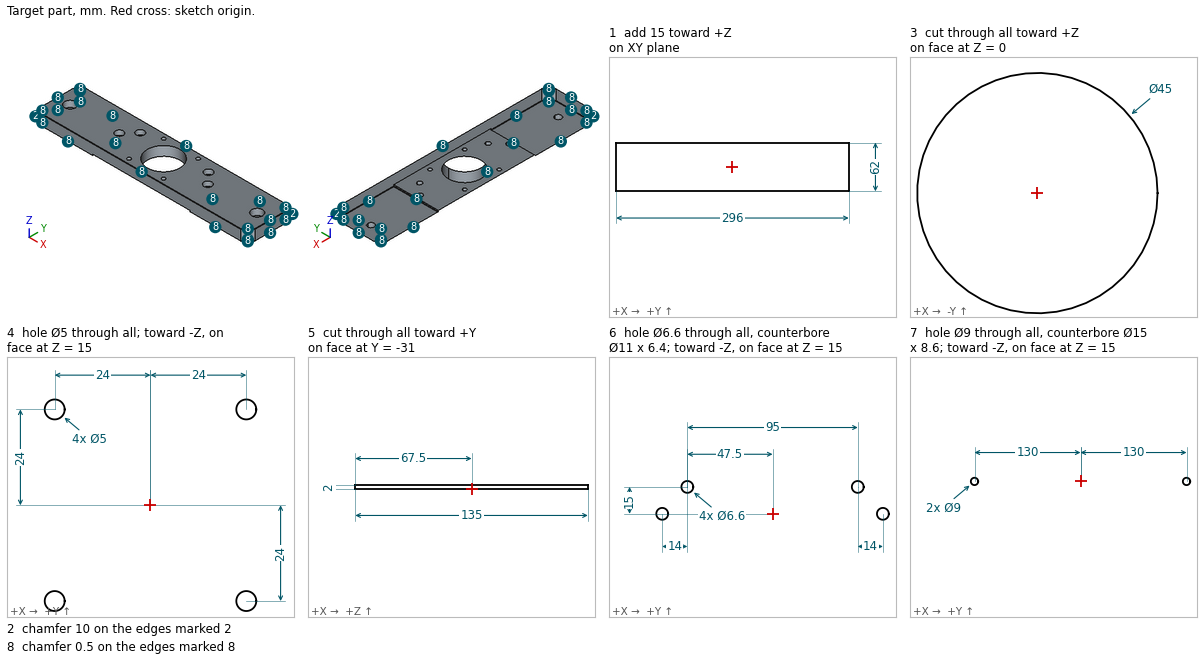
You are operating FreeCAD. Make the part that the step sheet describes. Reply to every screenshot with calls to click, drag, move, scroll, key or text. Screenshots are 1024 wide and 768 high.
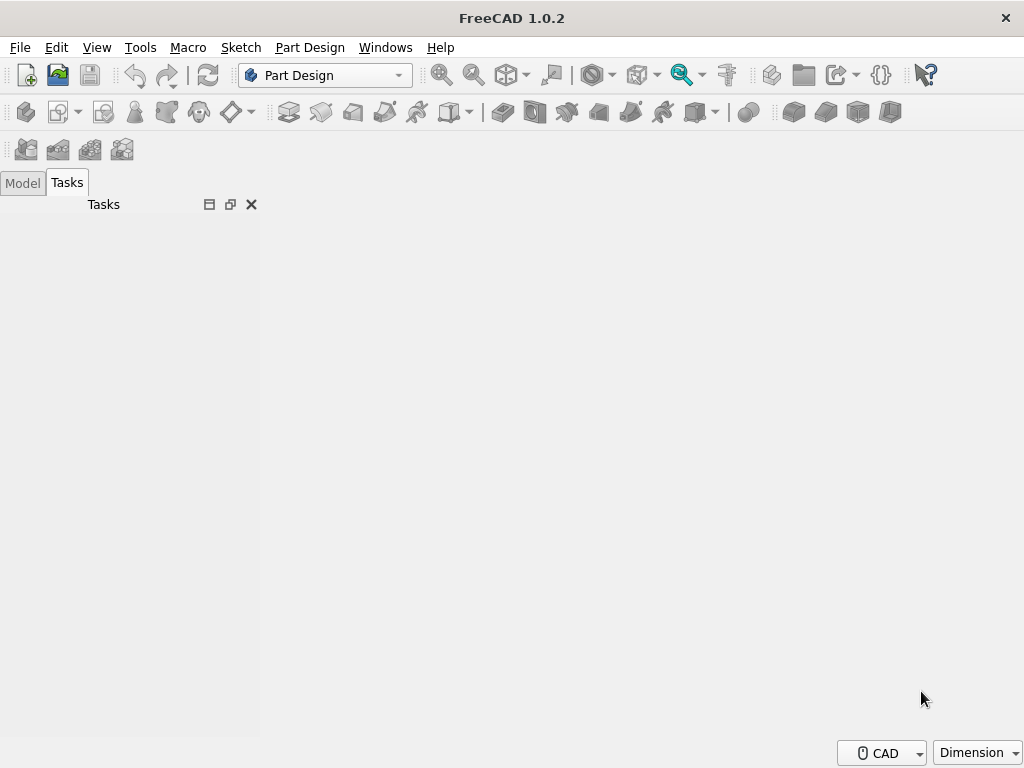
click(26, 76)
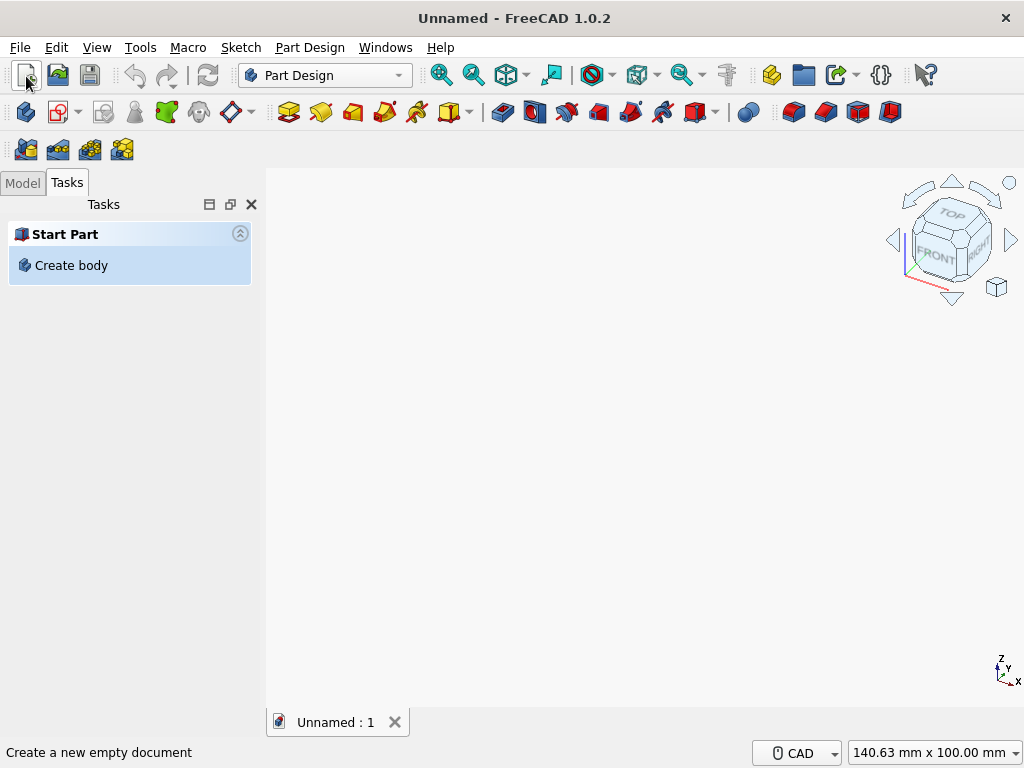
click(58, 112)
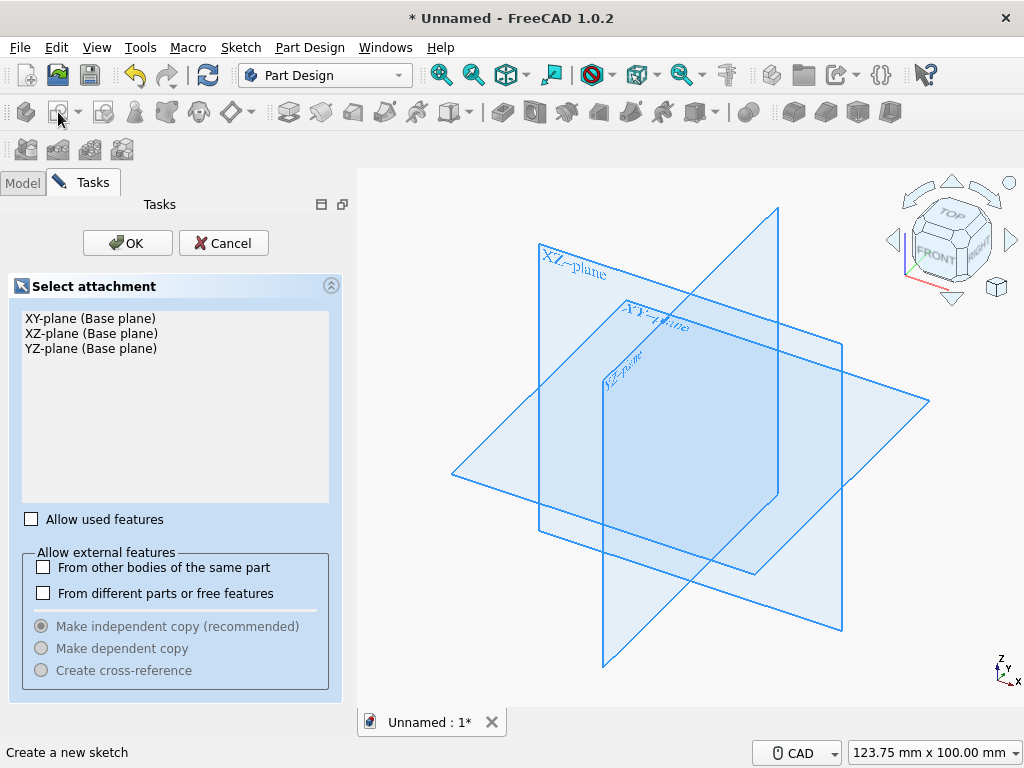
click(82, 318)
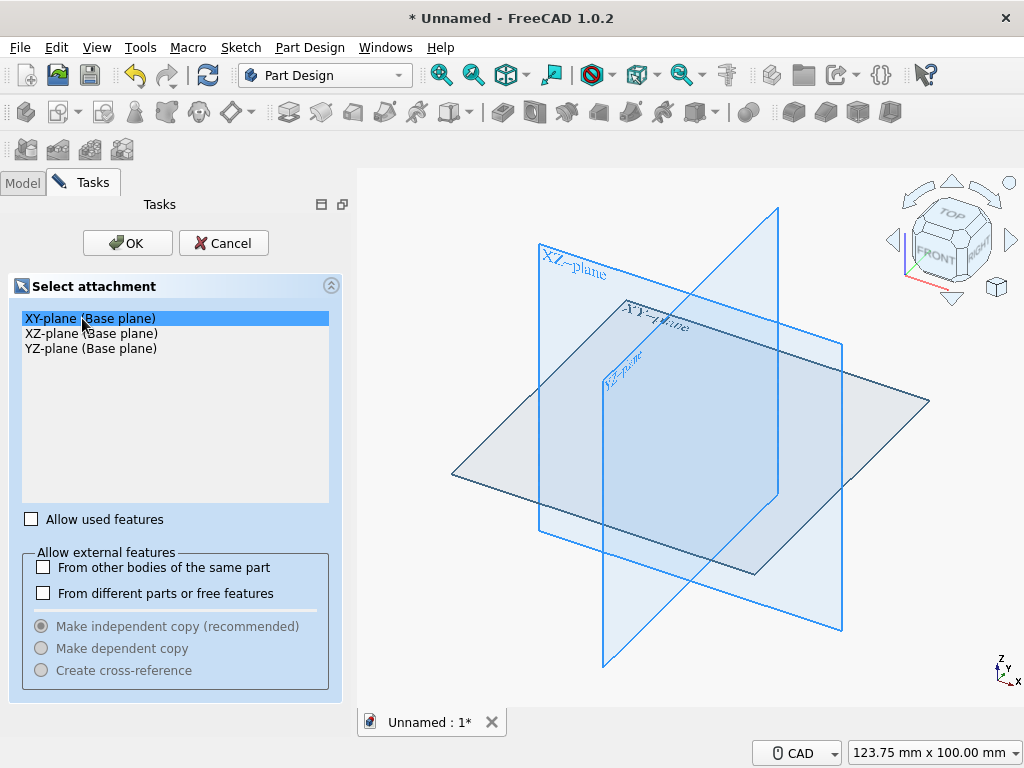
click(128, 243)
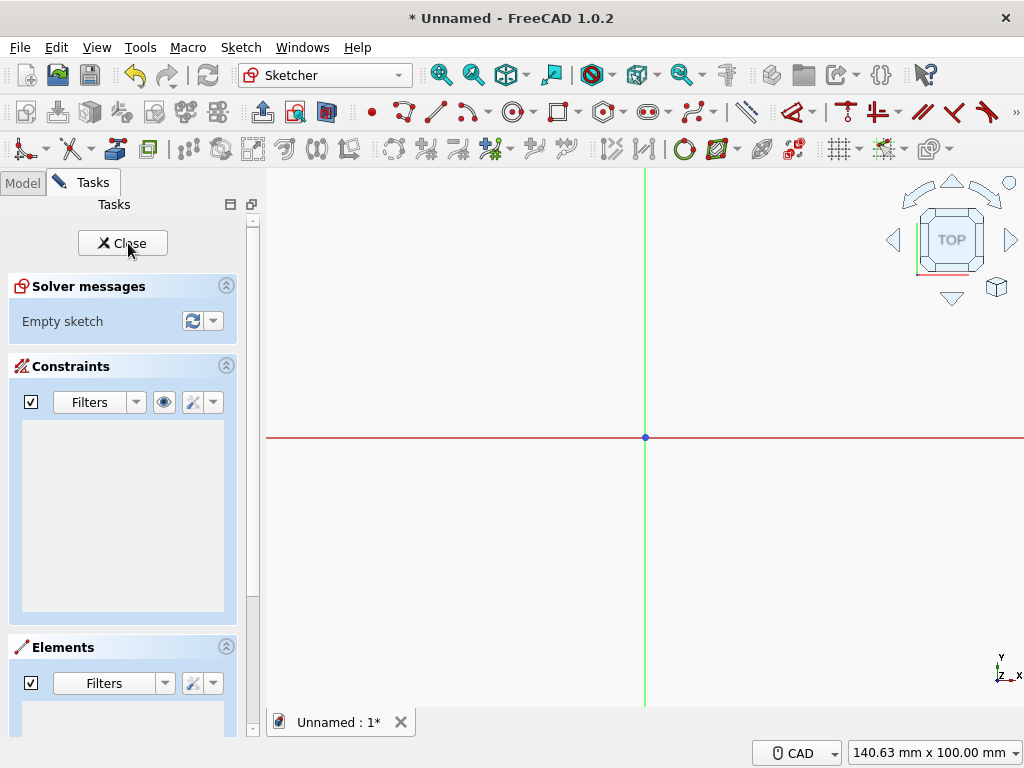
scroll(554, 438, down, 7)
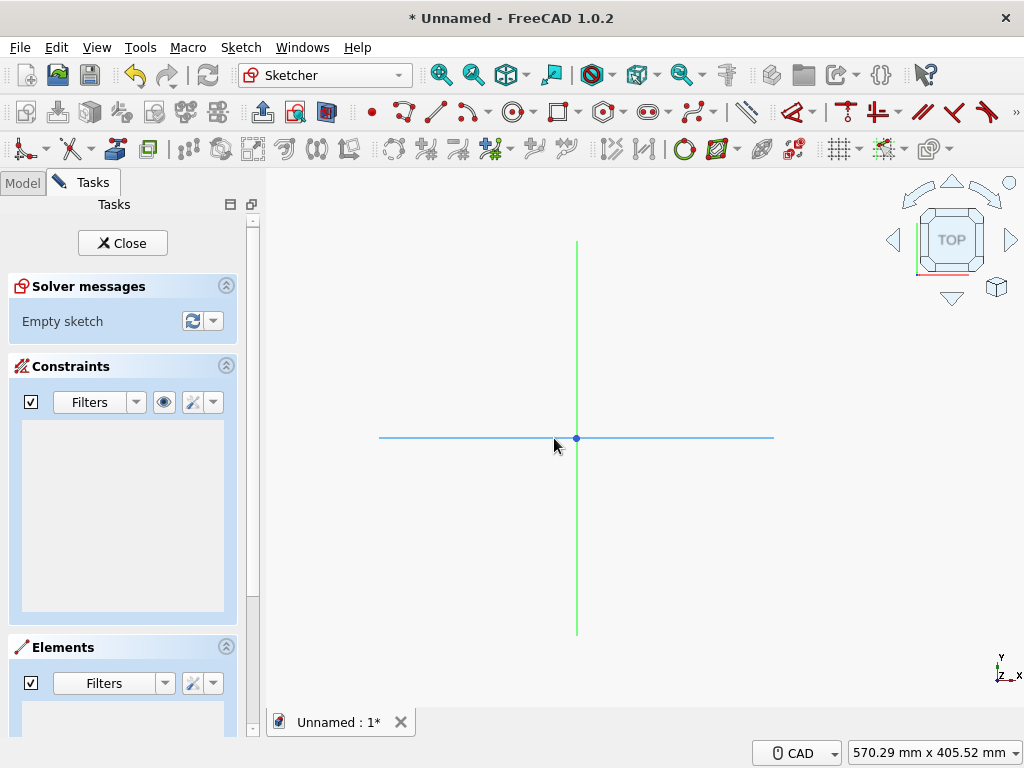
click(580, 112)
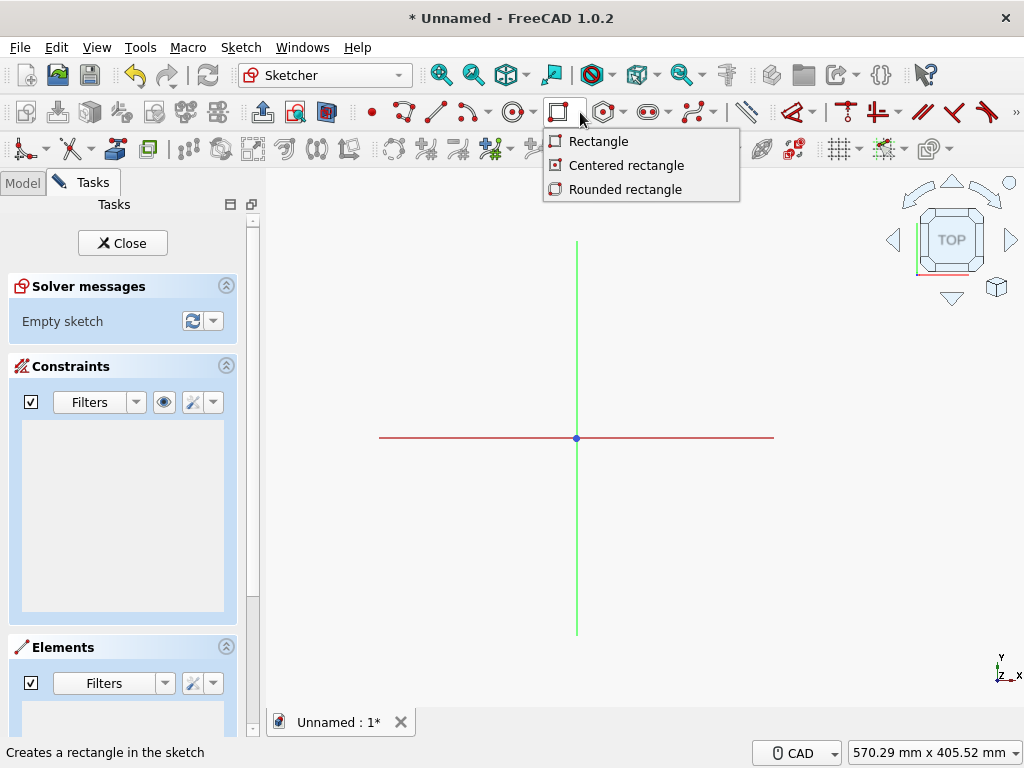
click(642, 165)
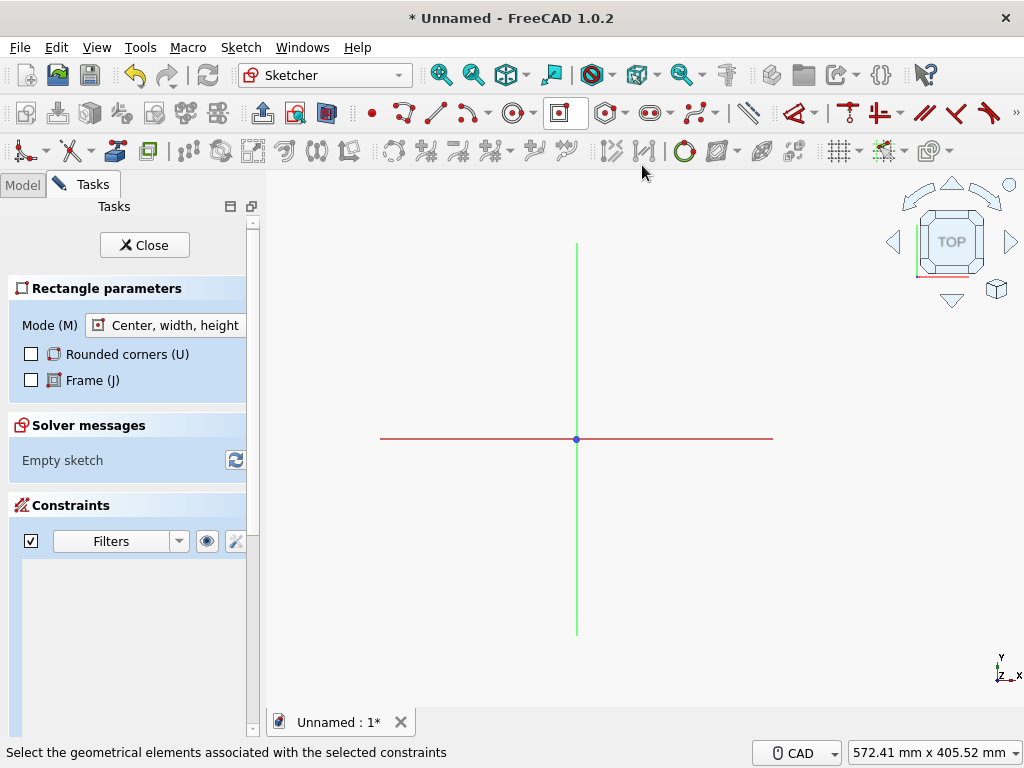
click(577, 439)
move(773, 398)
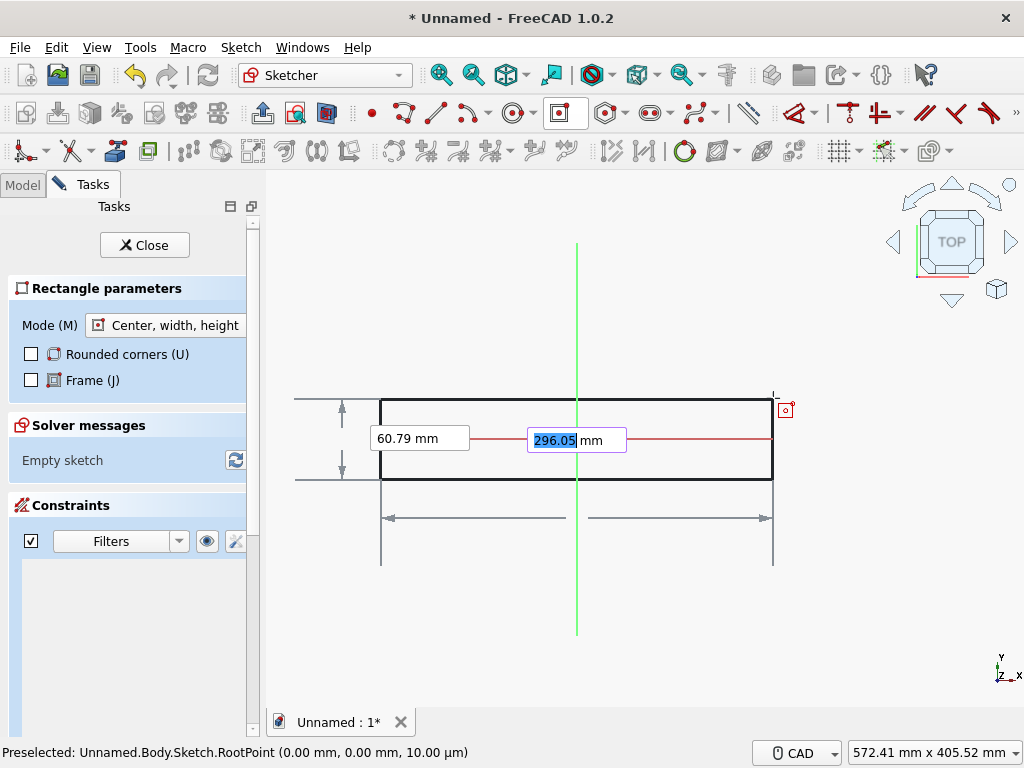
text(296)
key(Tab)
text(62)
key(Return)
key(Escape)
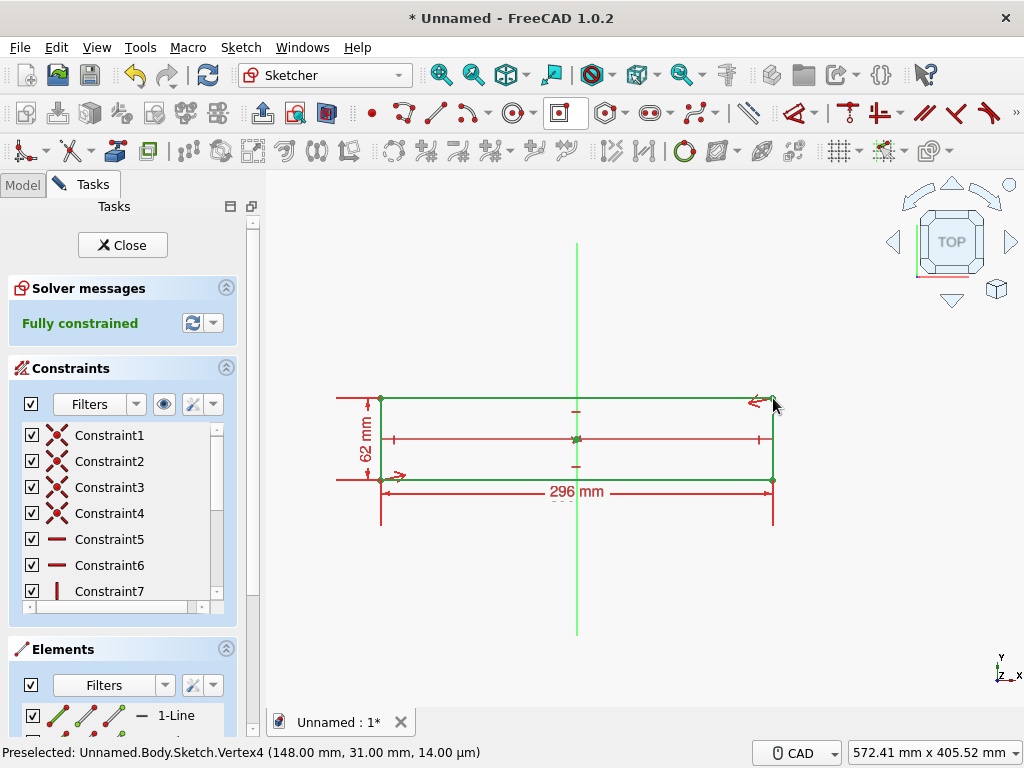
click(123, 245)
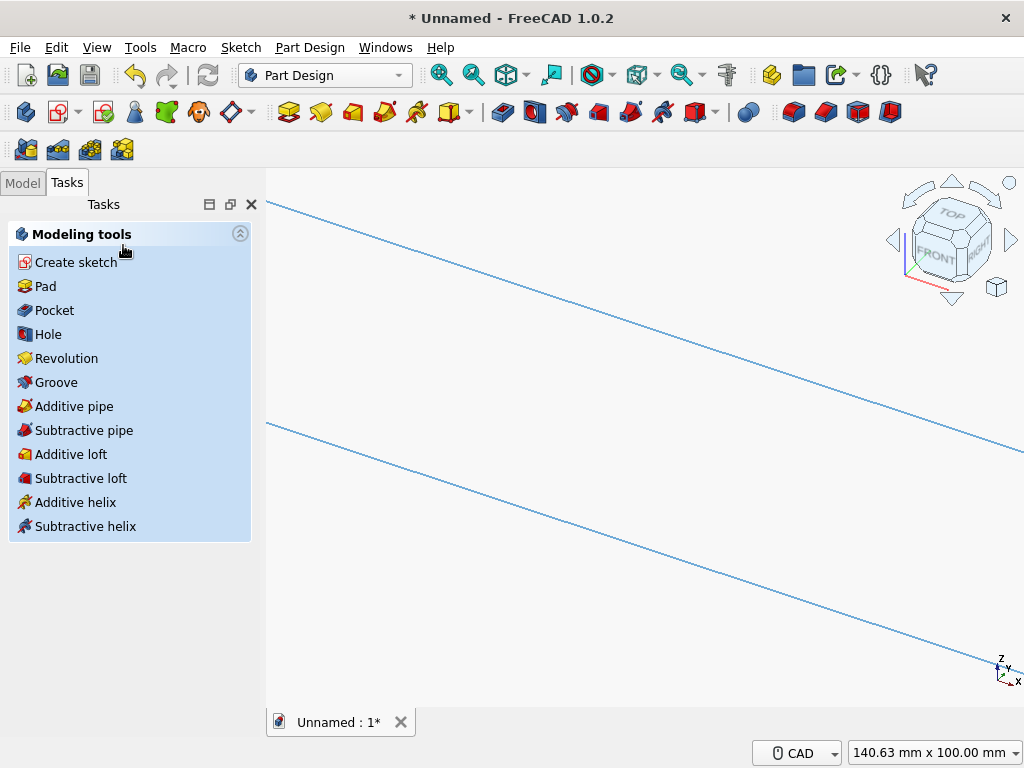
click(290, 112)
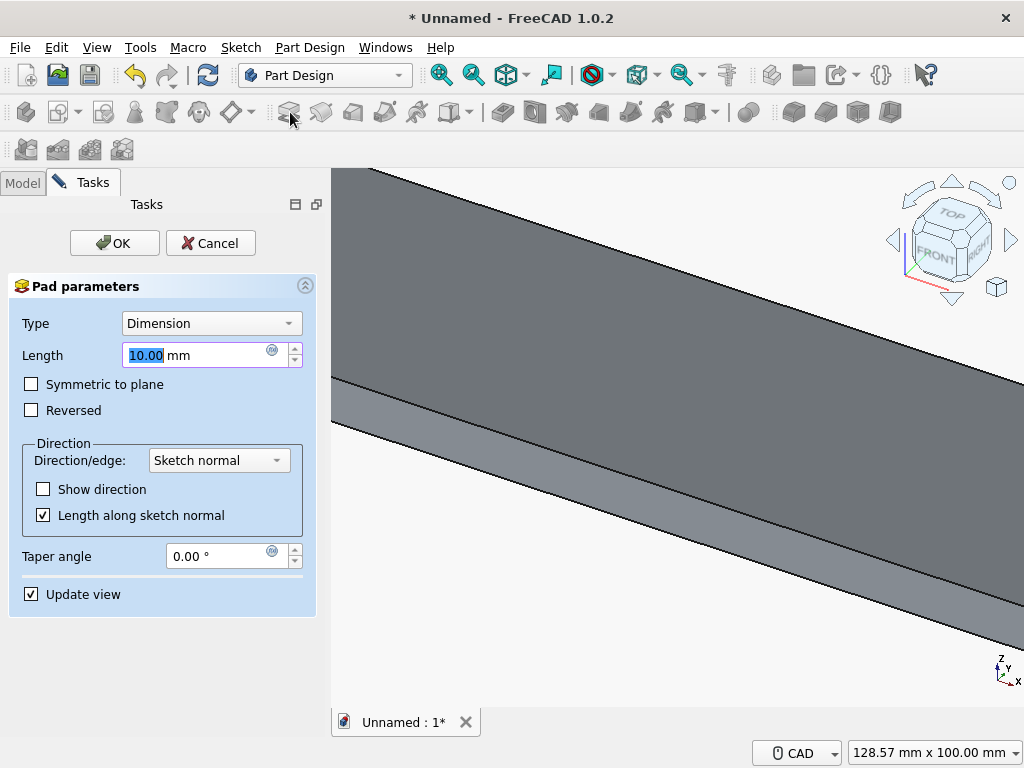
text(15)
key(Tab)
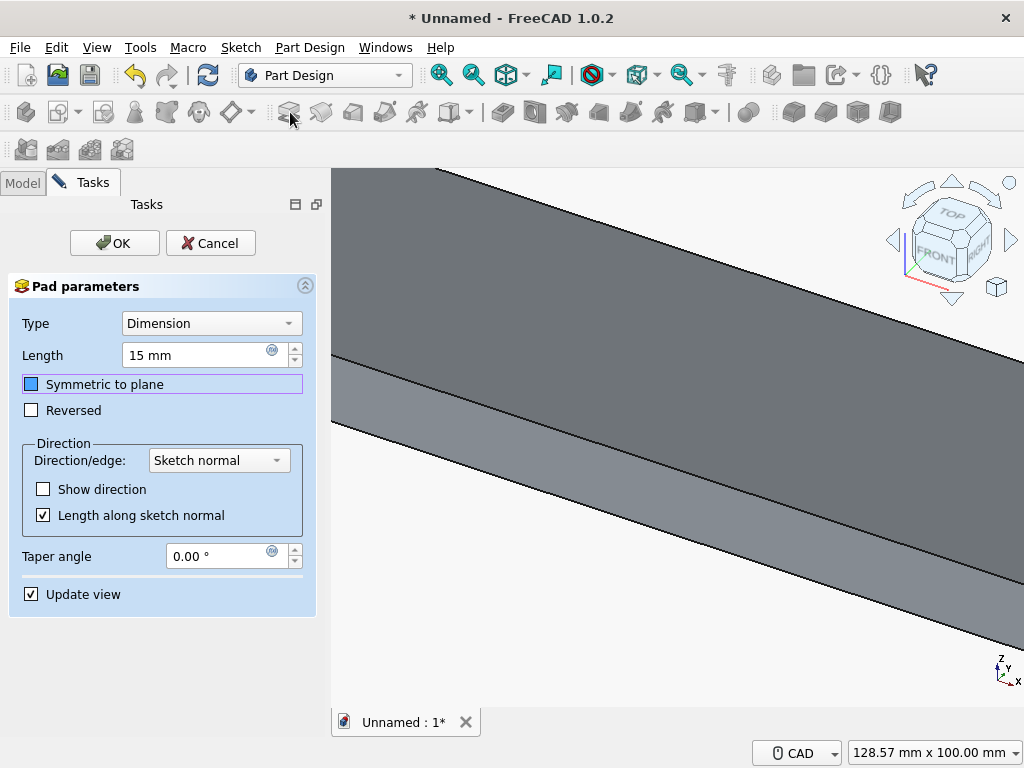
click(115, 243)